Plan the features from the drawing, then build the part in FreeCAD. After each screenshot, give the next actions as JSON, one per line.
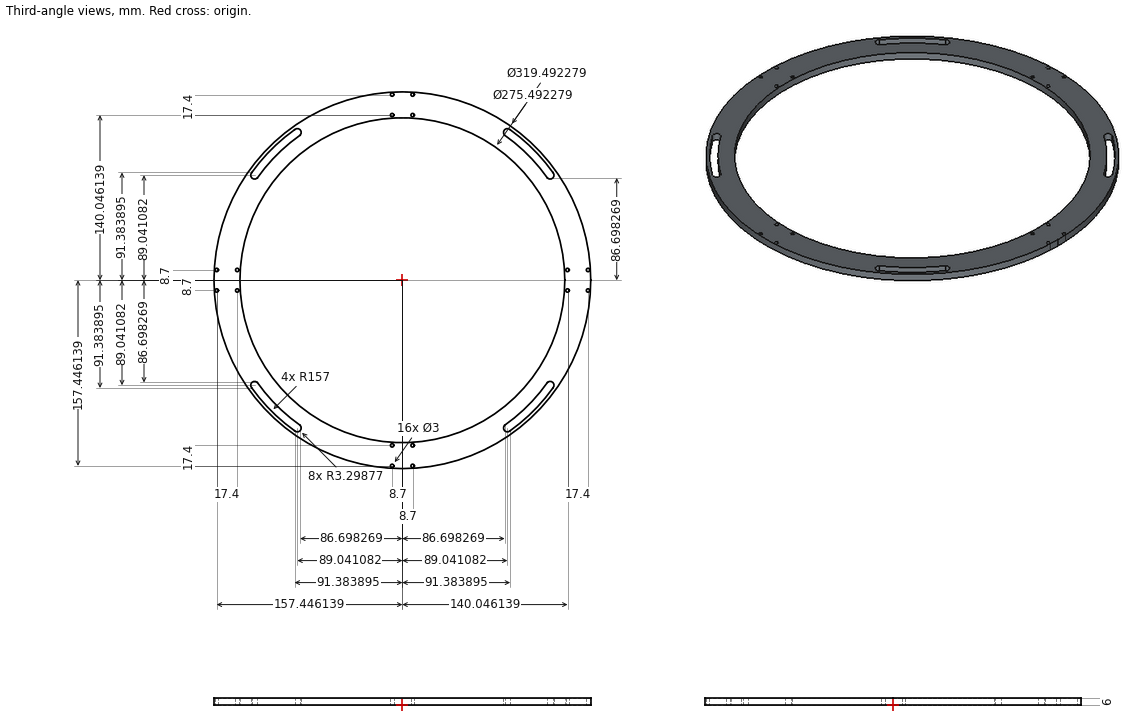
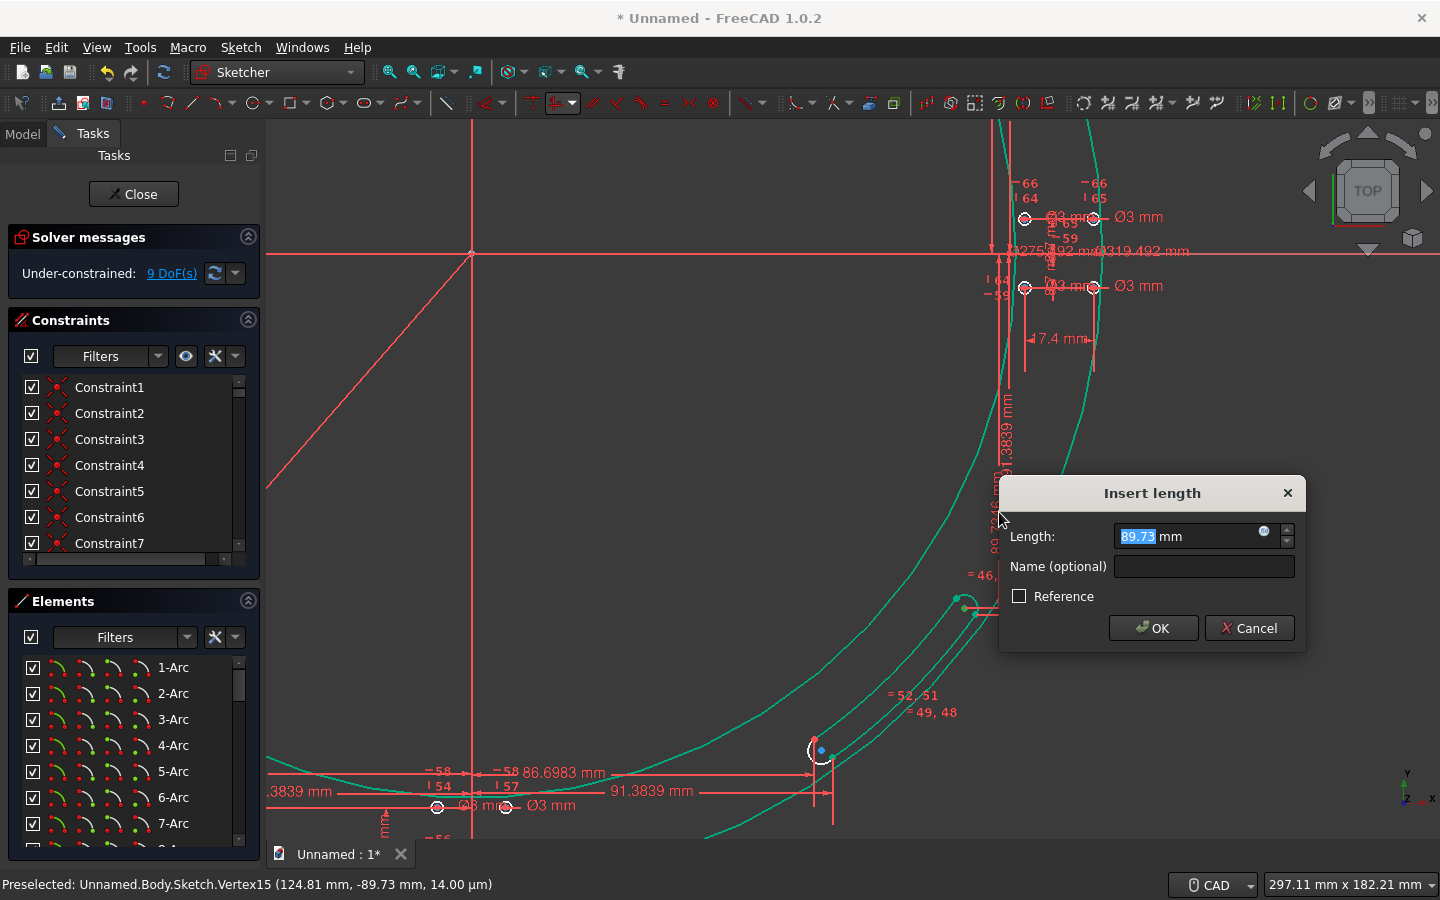
{"action": "type", "text": "89.041082"}
{"action": "key", "text": "Return"}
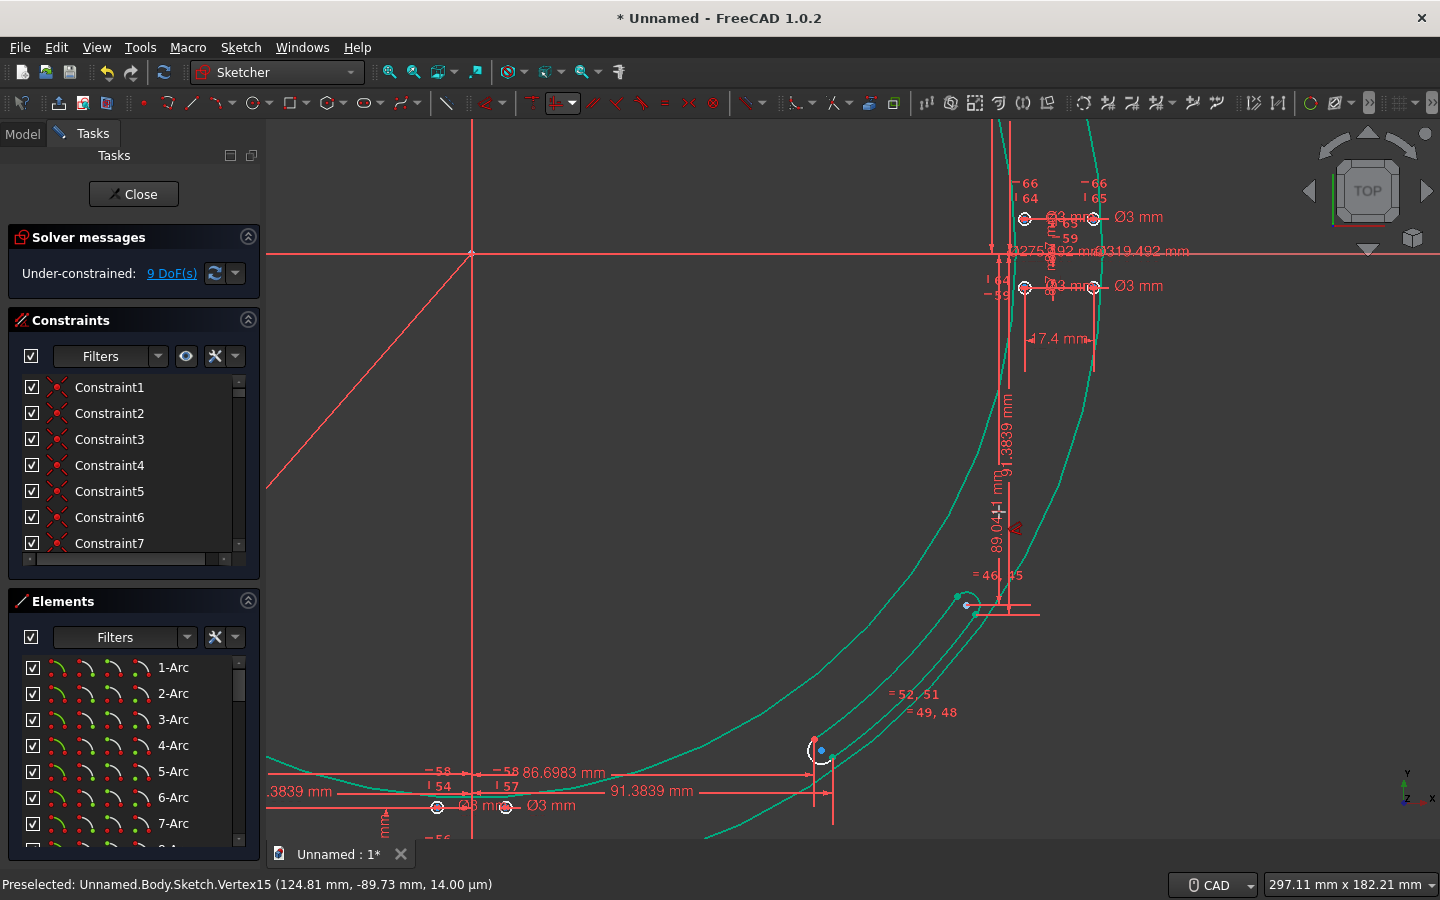
{"action": "left_click", "coordinate": [821, 751]}
{"action": "left_click", "coordinate": [727, 785]}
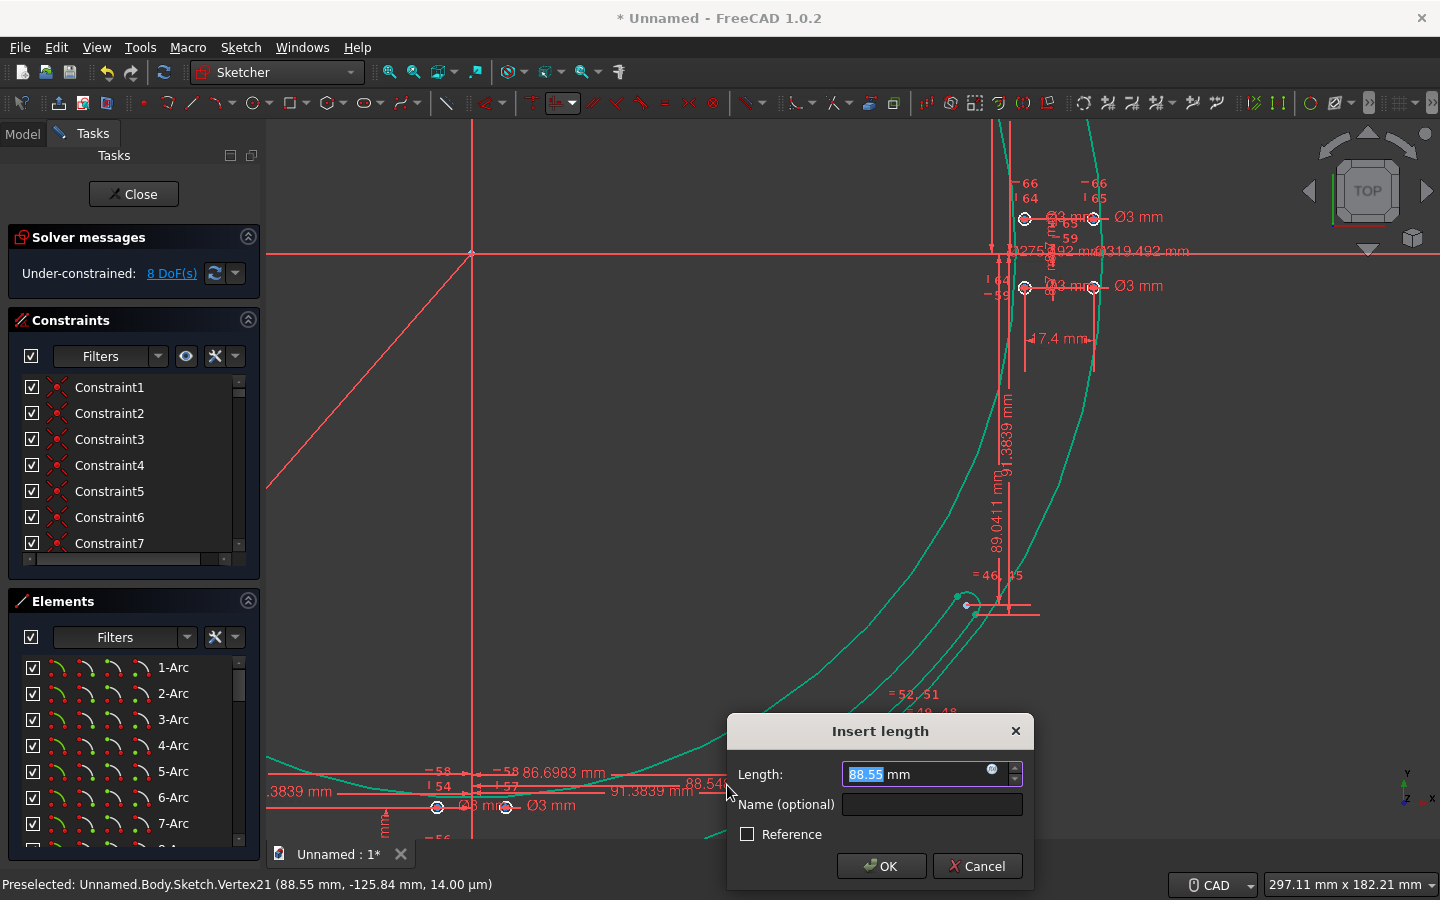
{"action": "type", "text": "89.041082"}
{"action": "key", "text": "Return"}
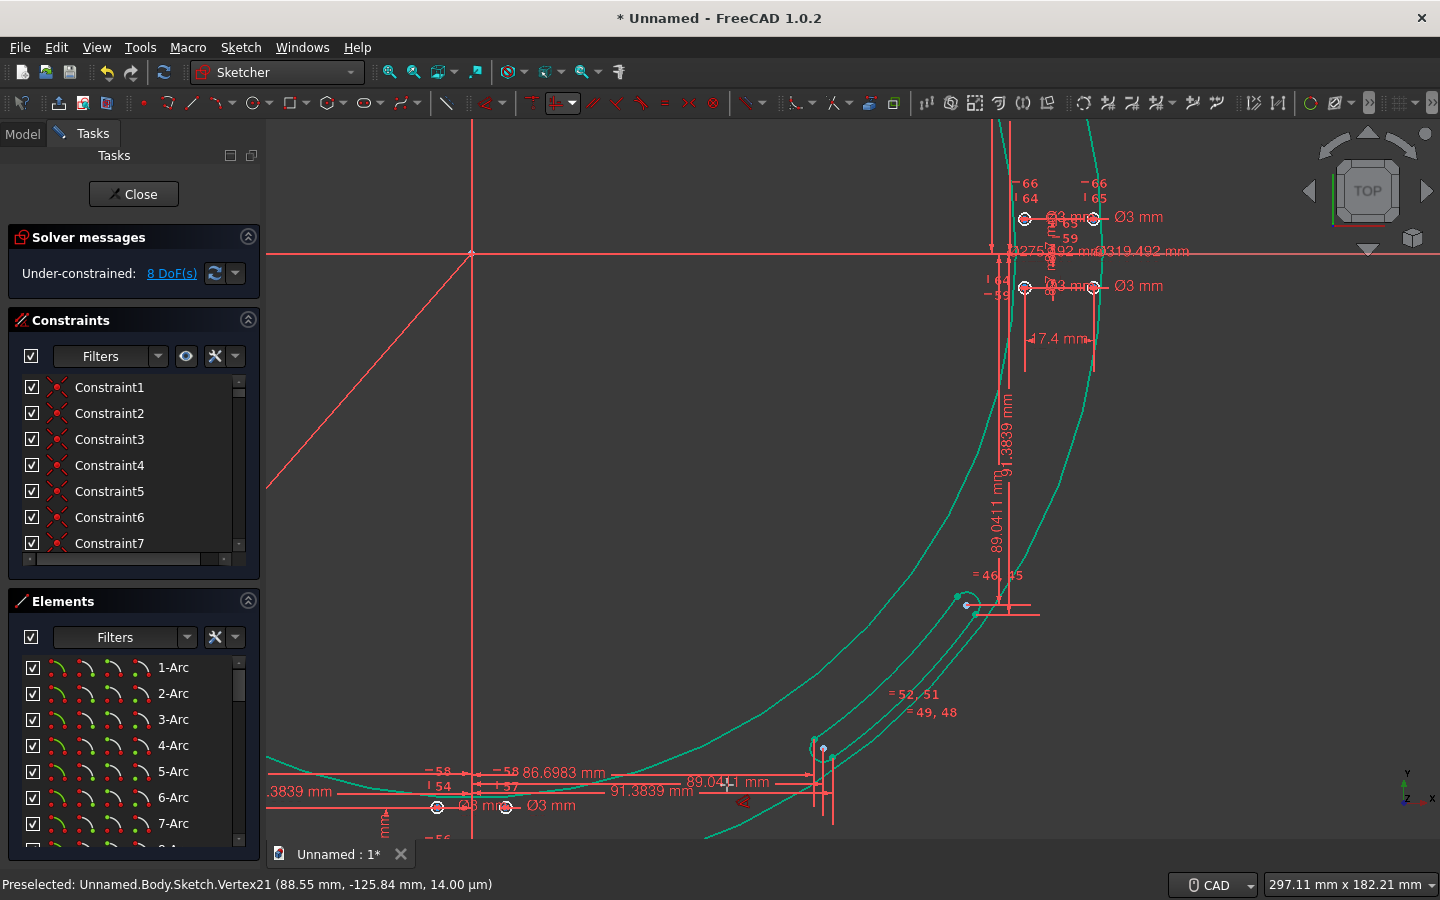
{"action": "scroll", "coordinate": [967, 610], "scroll_direction": "down", "scroll_amount": 5}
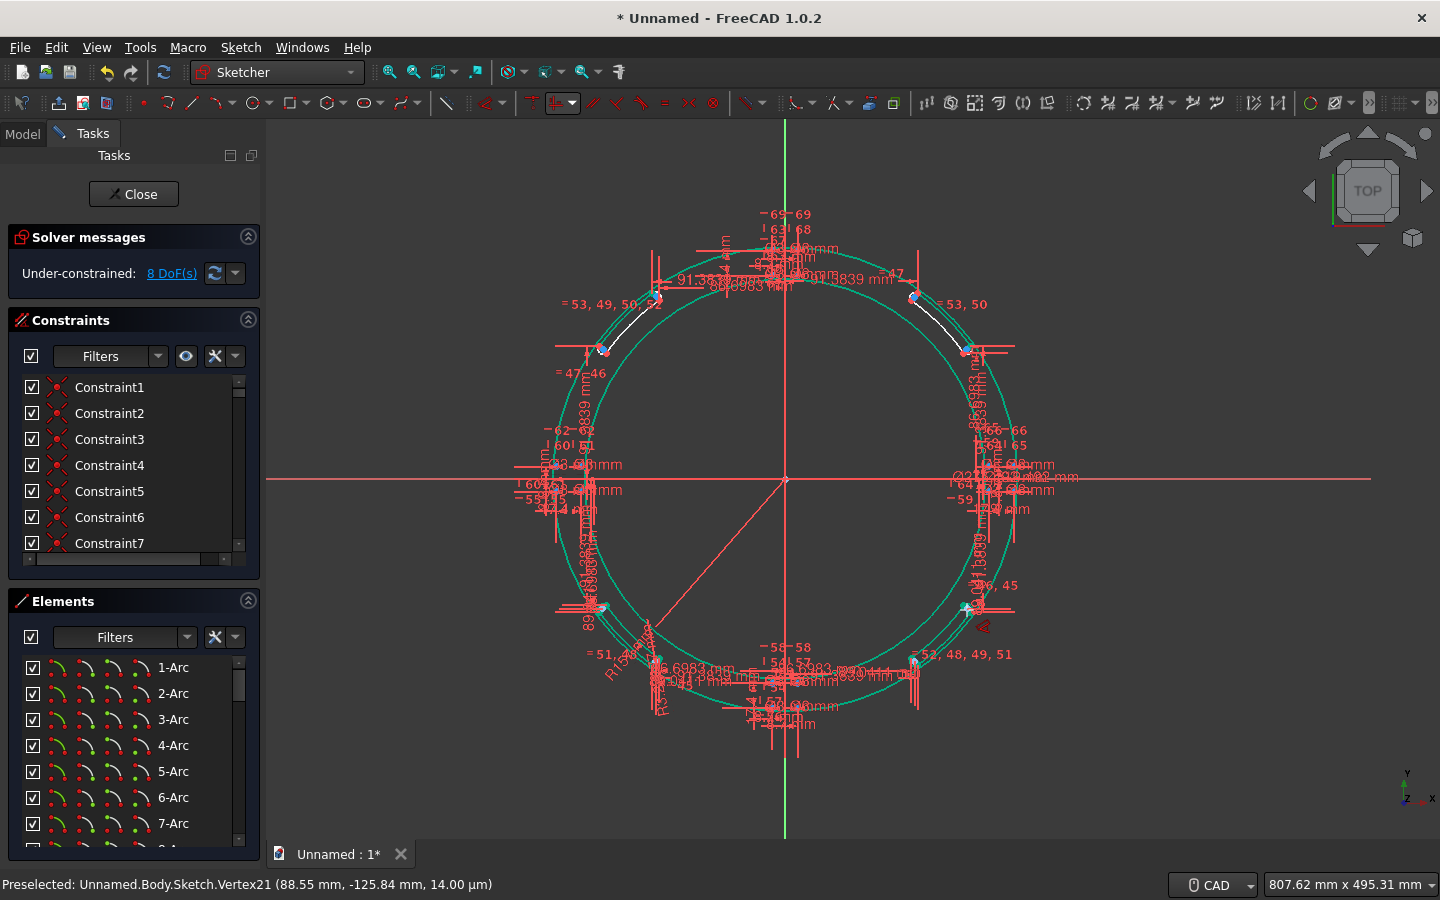
{"action": "scroll", "coordinate": [603, 350], "scroll_direction": "up", "scroll_amount": 5}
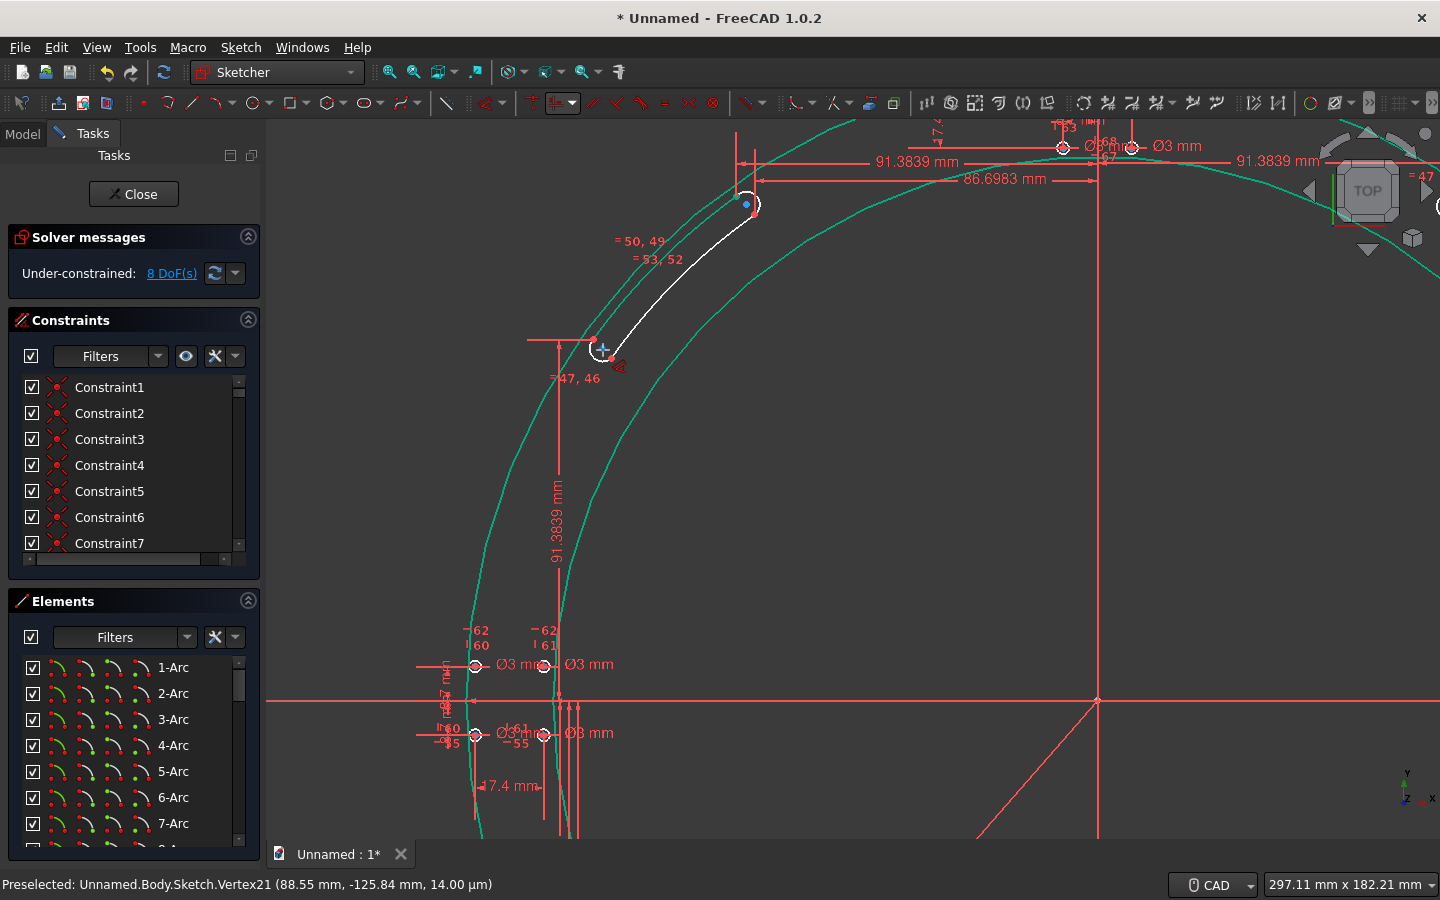
{"action": "left_click", "coordinate": [603, 348]}
{"action": "left_click", "coordinate": [569, 444]}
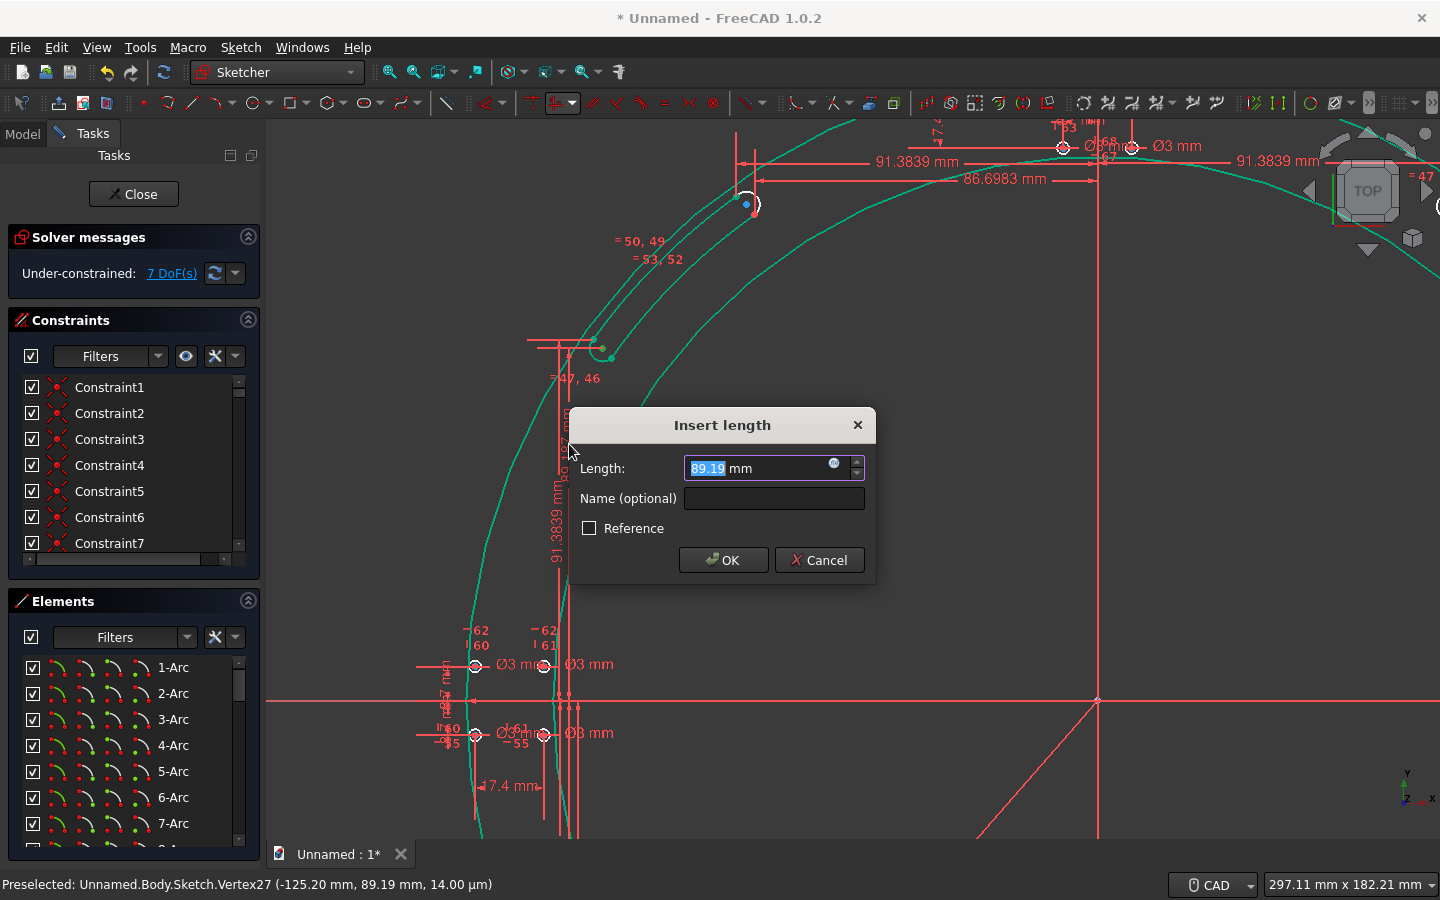
{"action": "type", "text": "89.041082"}
{"action": "key", "text": "Return"}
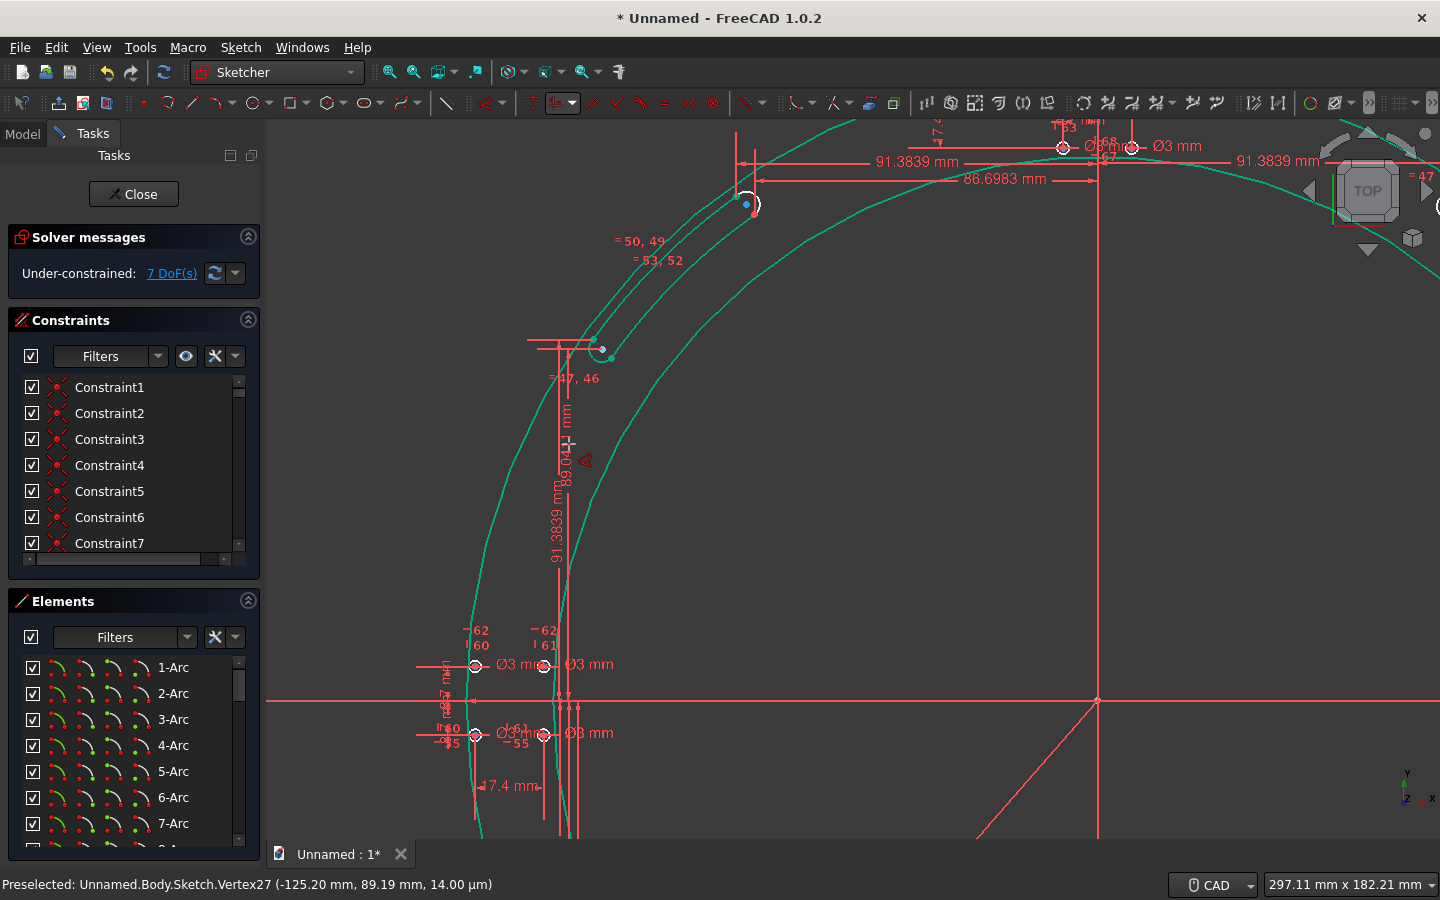
{"action": "left_click", "coordinate": [747, 205]}
{"action": "left_click", "coordinate": [841, 171]}